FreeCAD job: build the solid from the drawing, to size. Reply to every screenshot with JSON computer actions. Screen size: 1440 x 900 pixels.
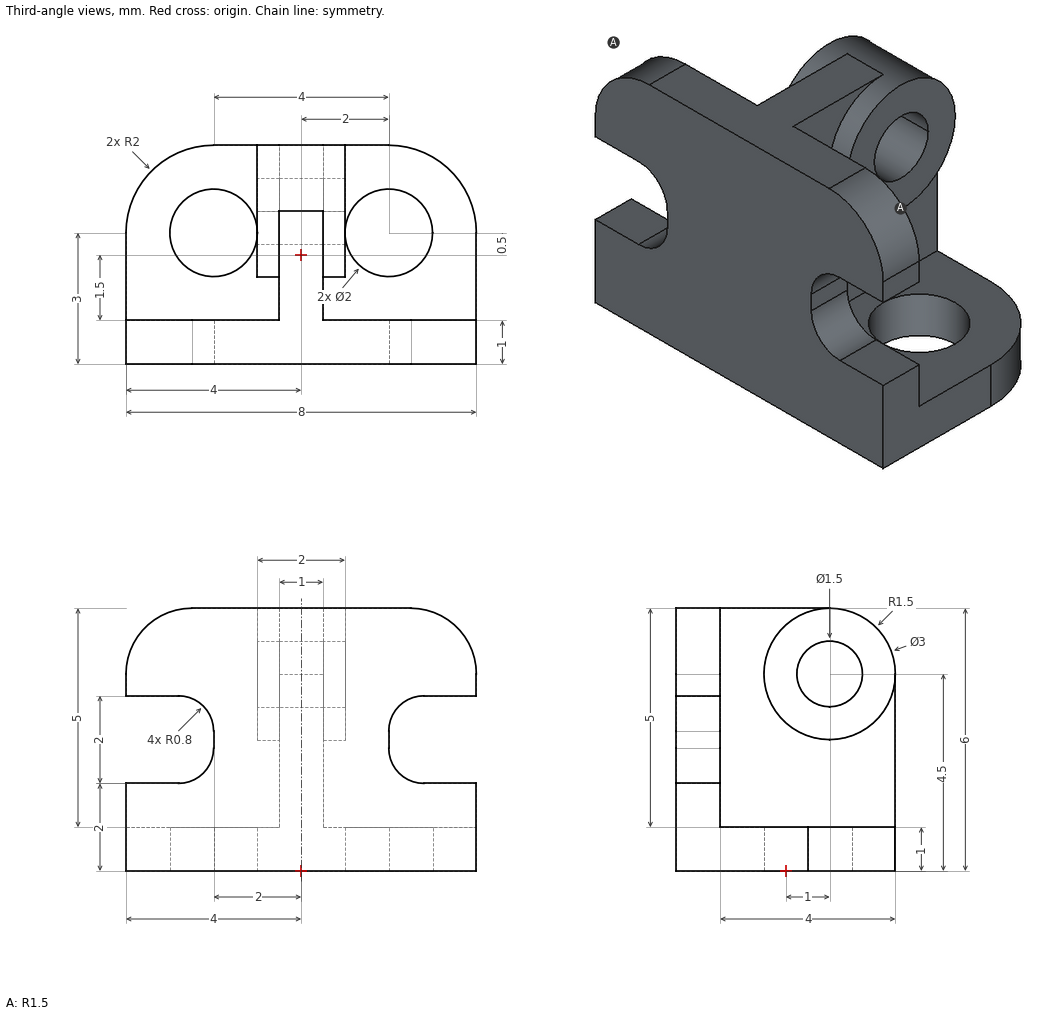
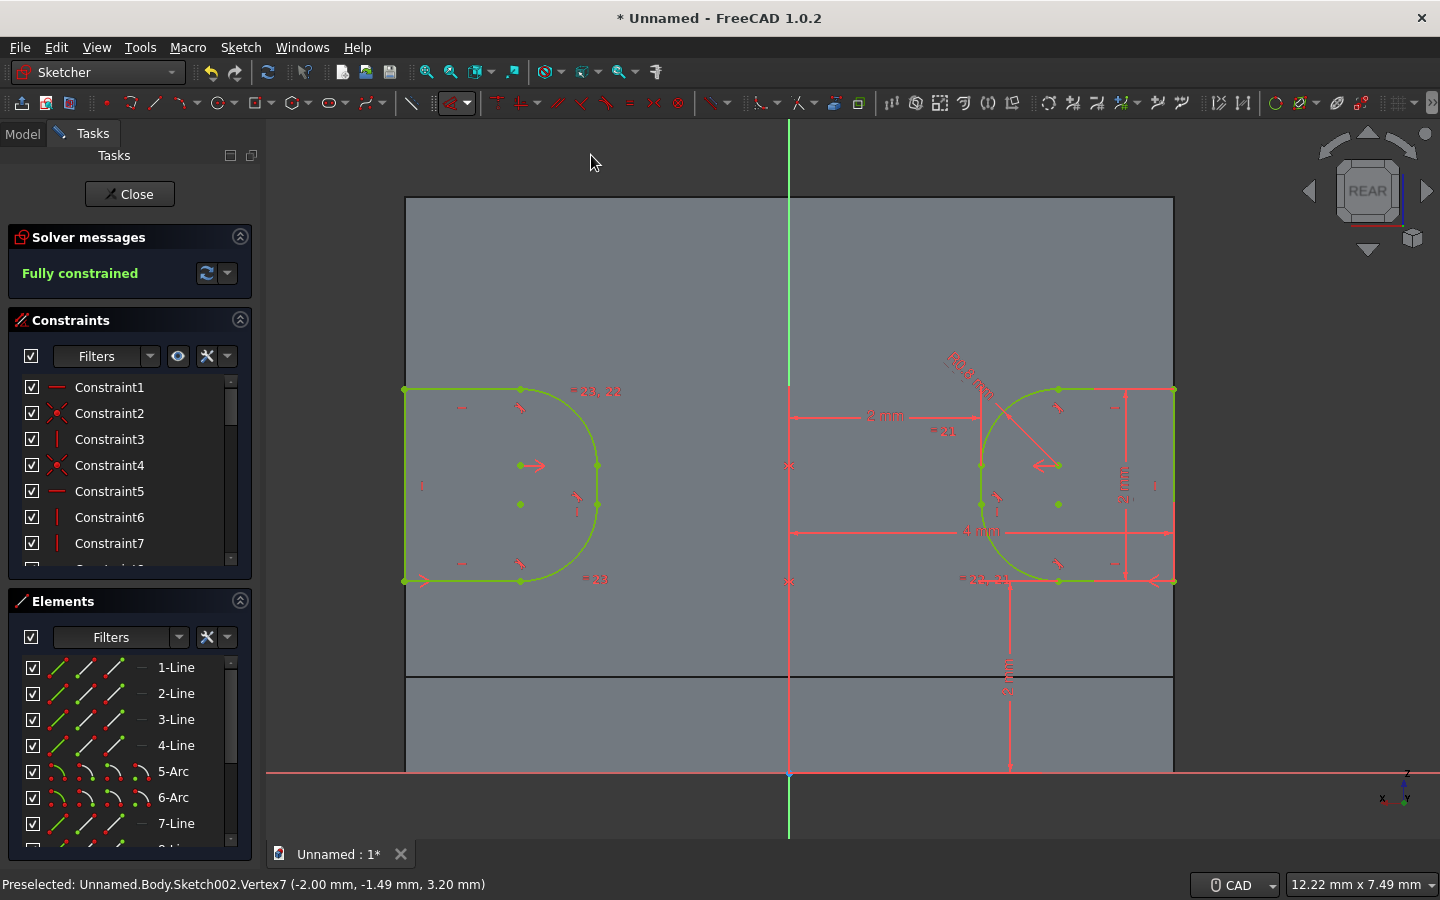
{"action": "left_click", "coordinate": [130, 194]}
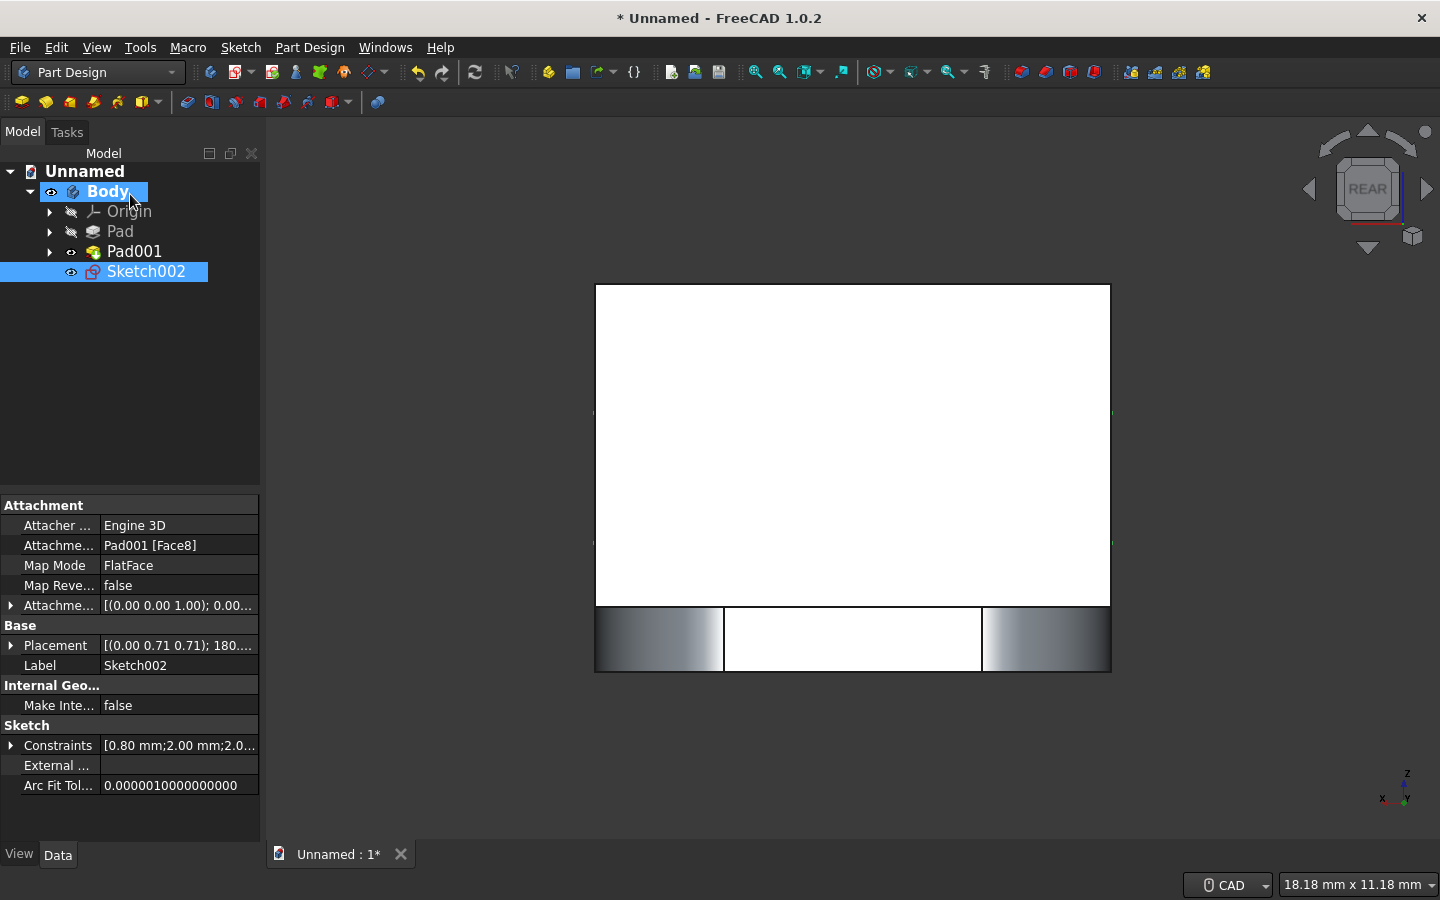
{"action": "left_click", "coordinate": [188, 102]}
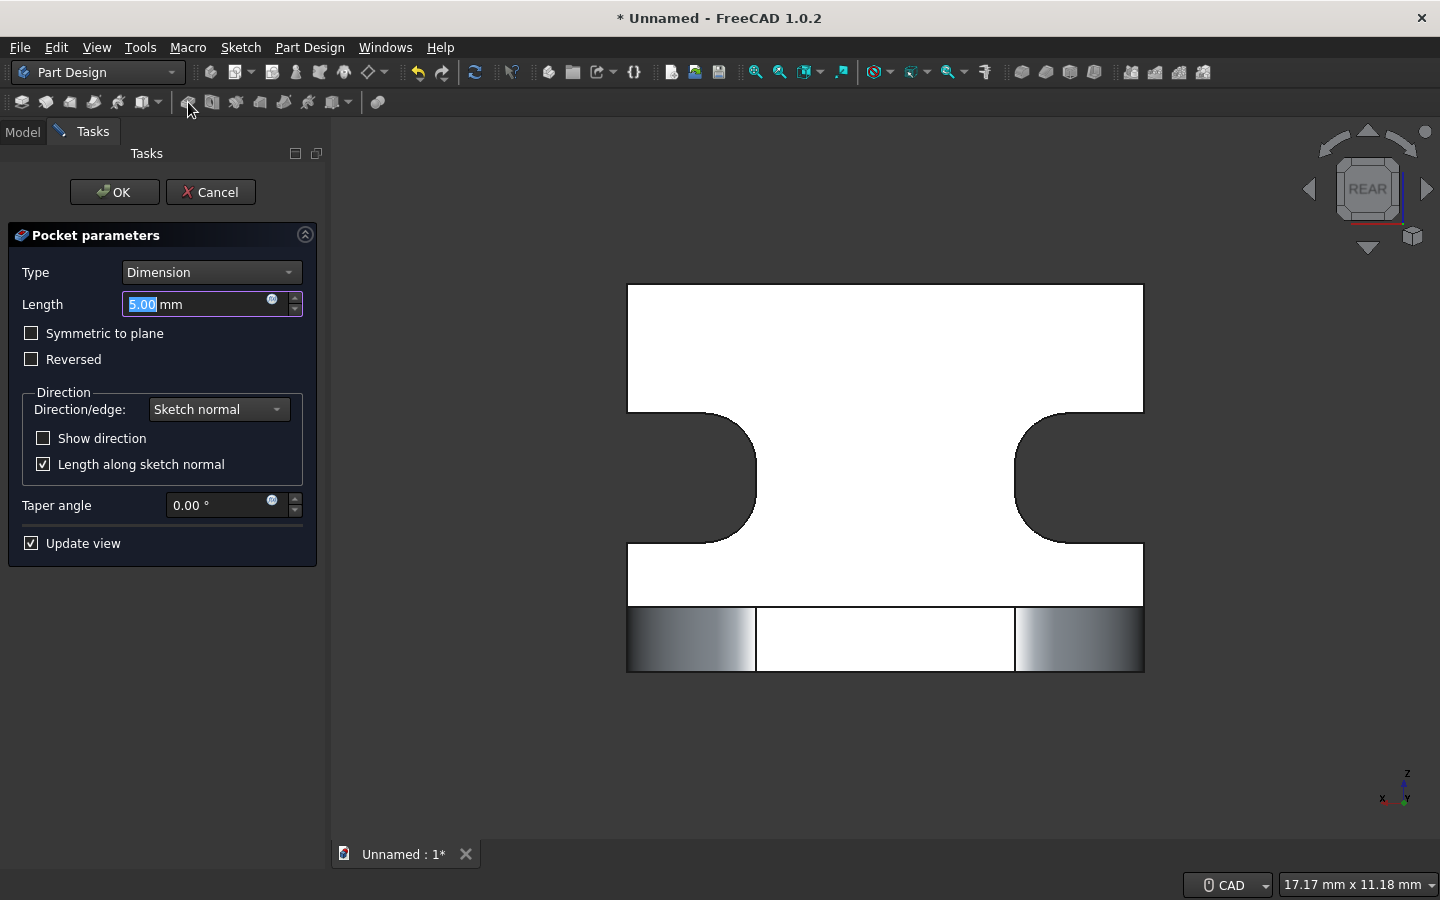
{"action": "left_click", "coordinate": [212, 272]}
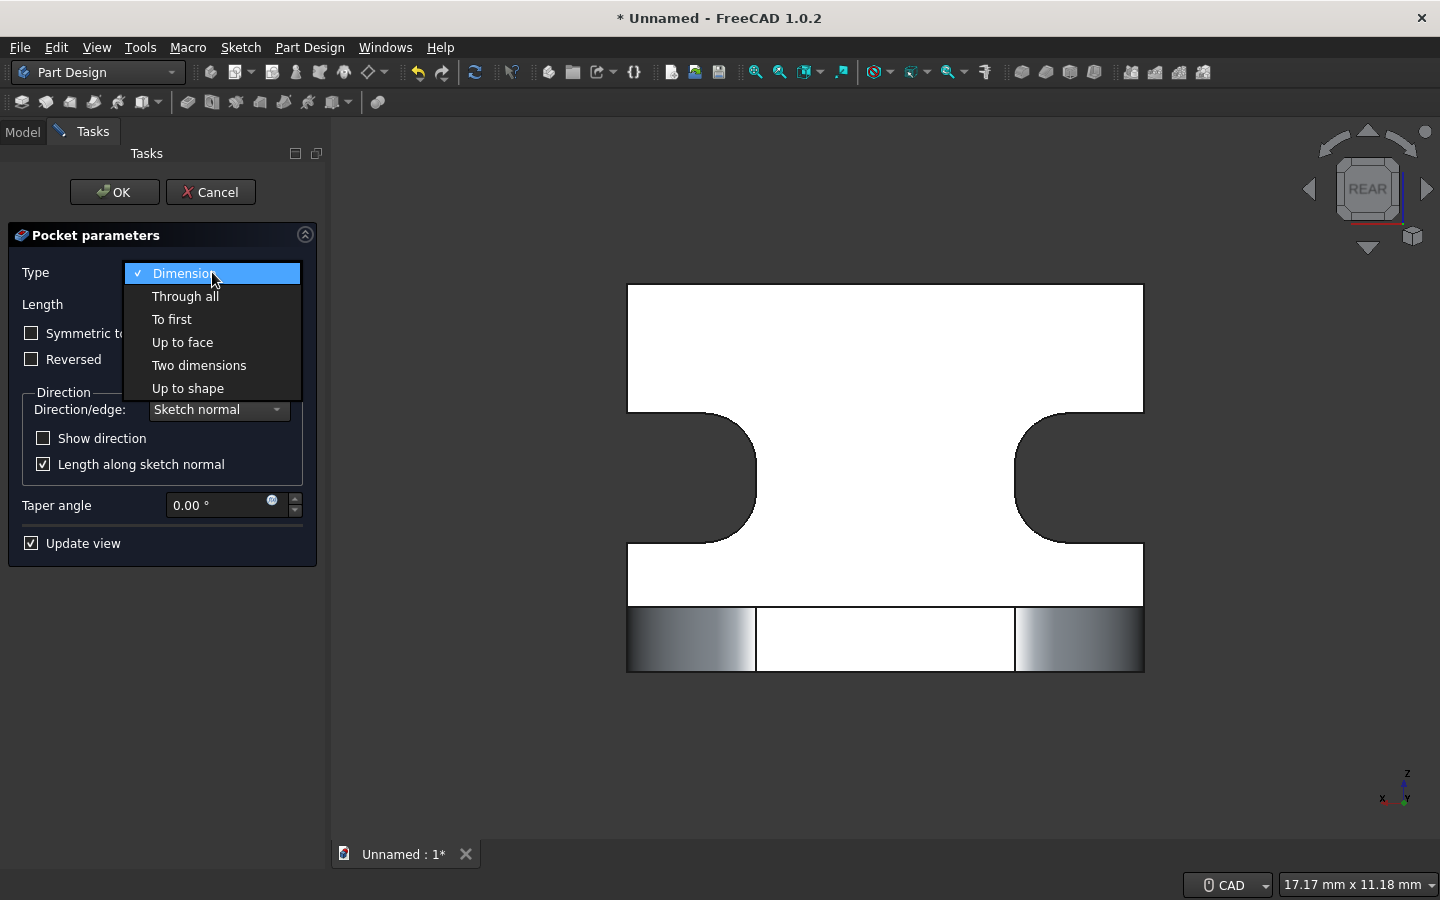
{"action": "left_click", "coordinate": [212, 296]}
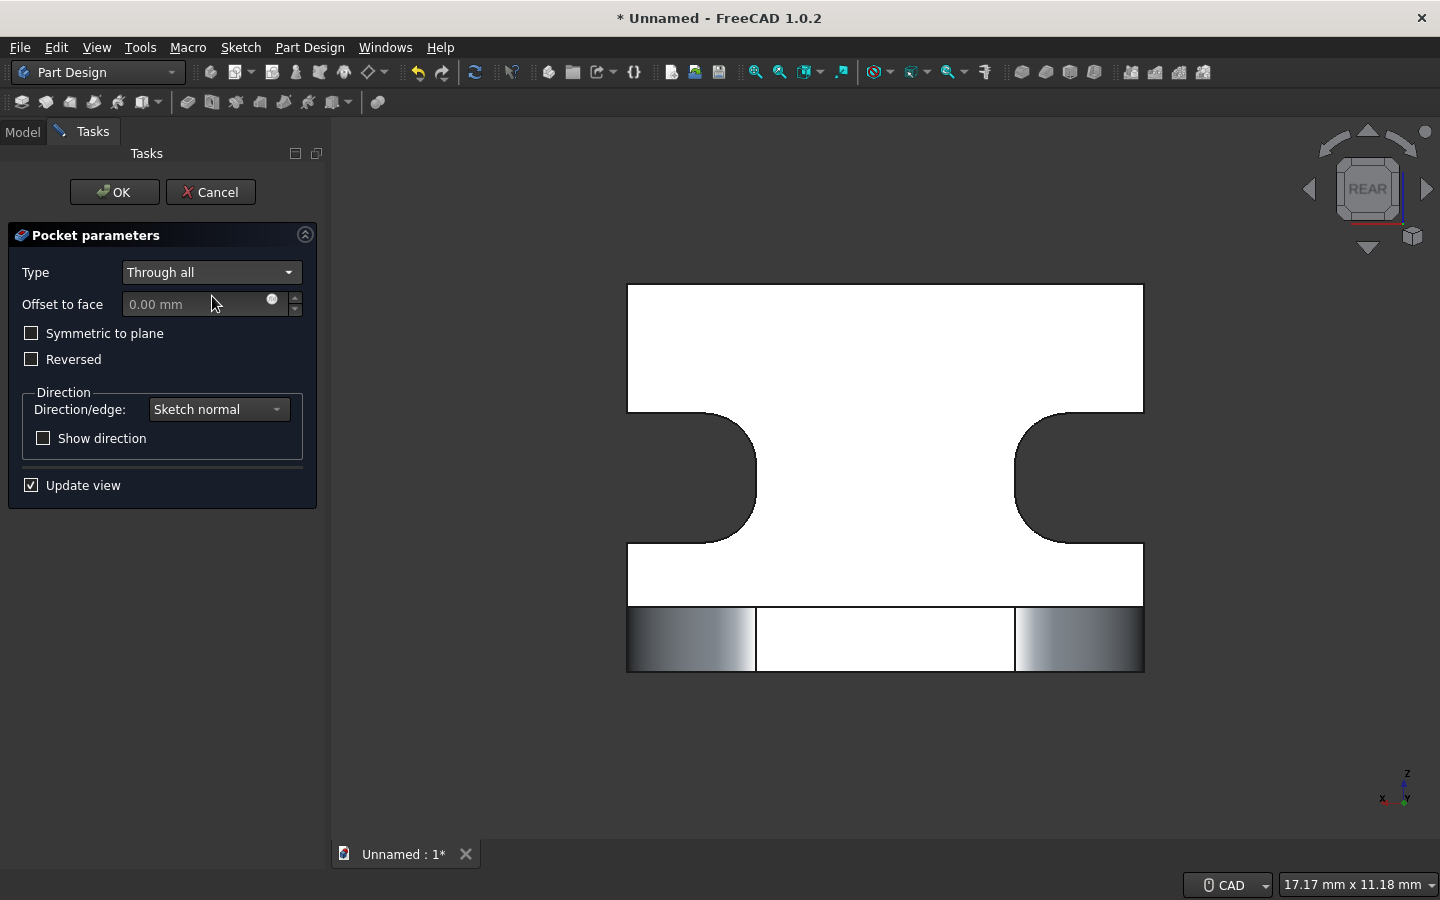
{"action": "left_click", "coordinate": [115, 192]}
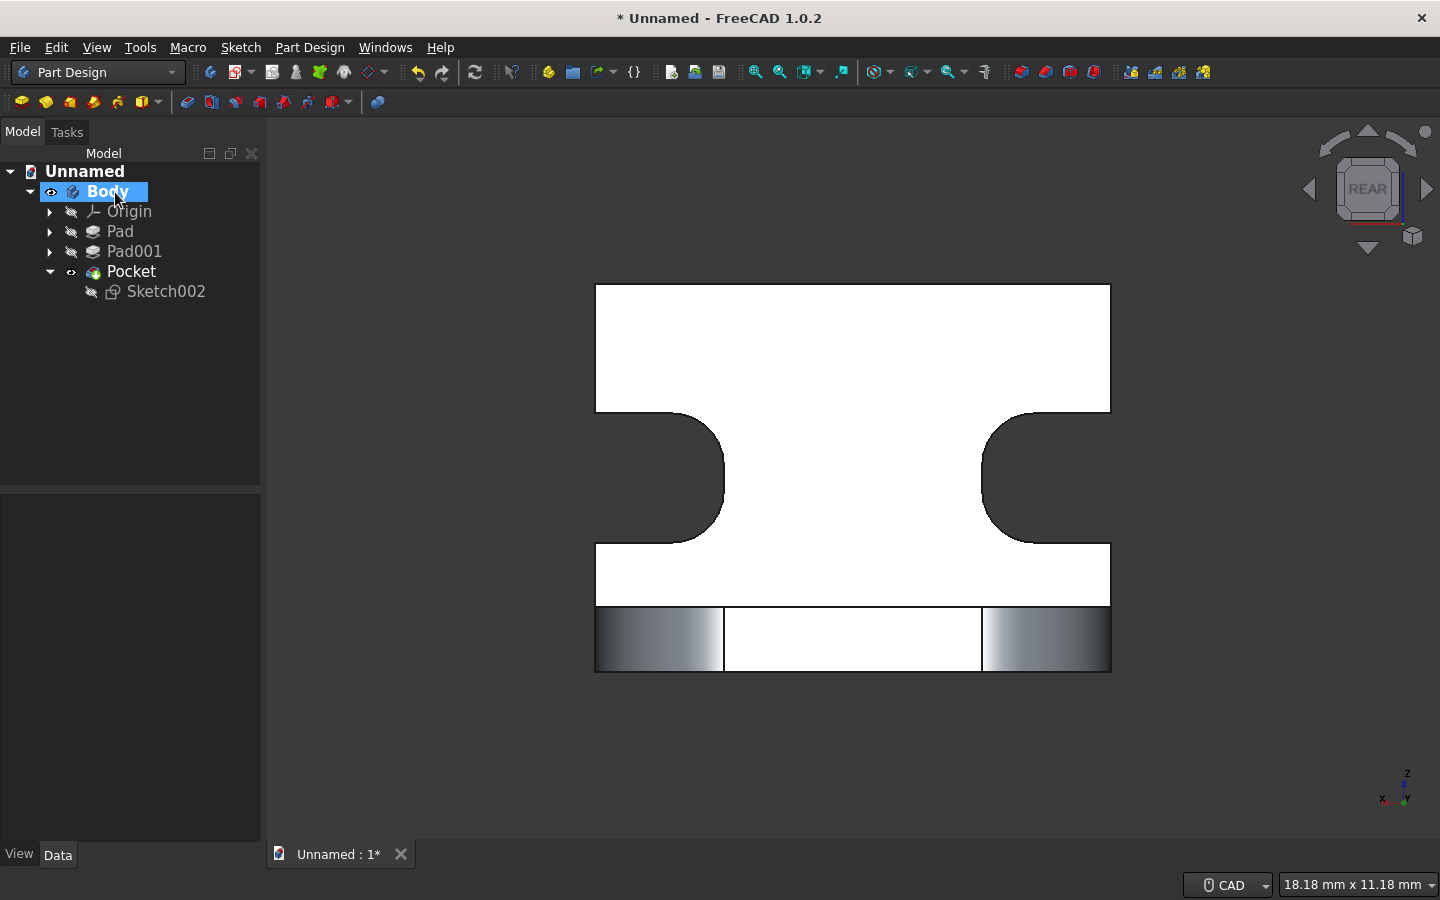
{"action": "left_click", "coordinate": [236, 72]}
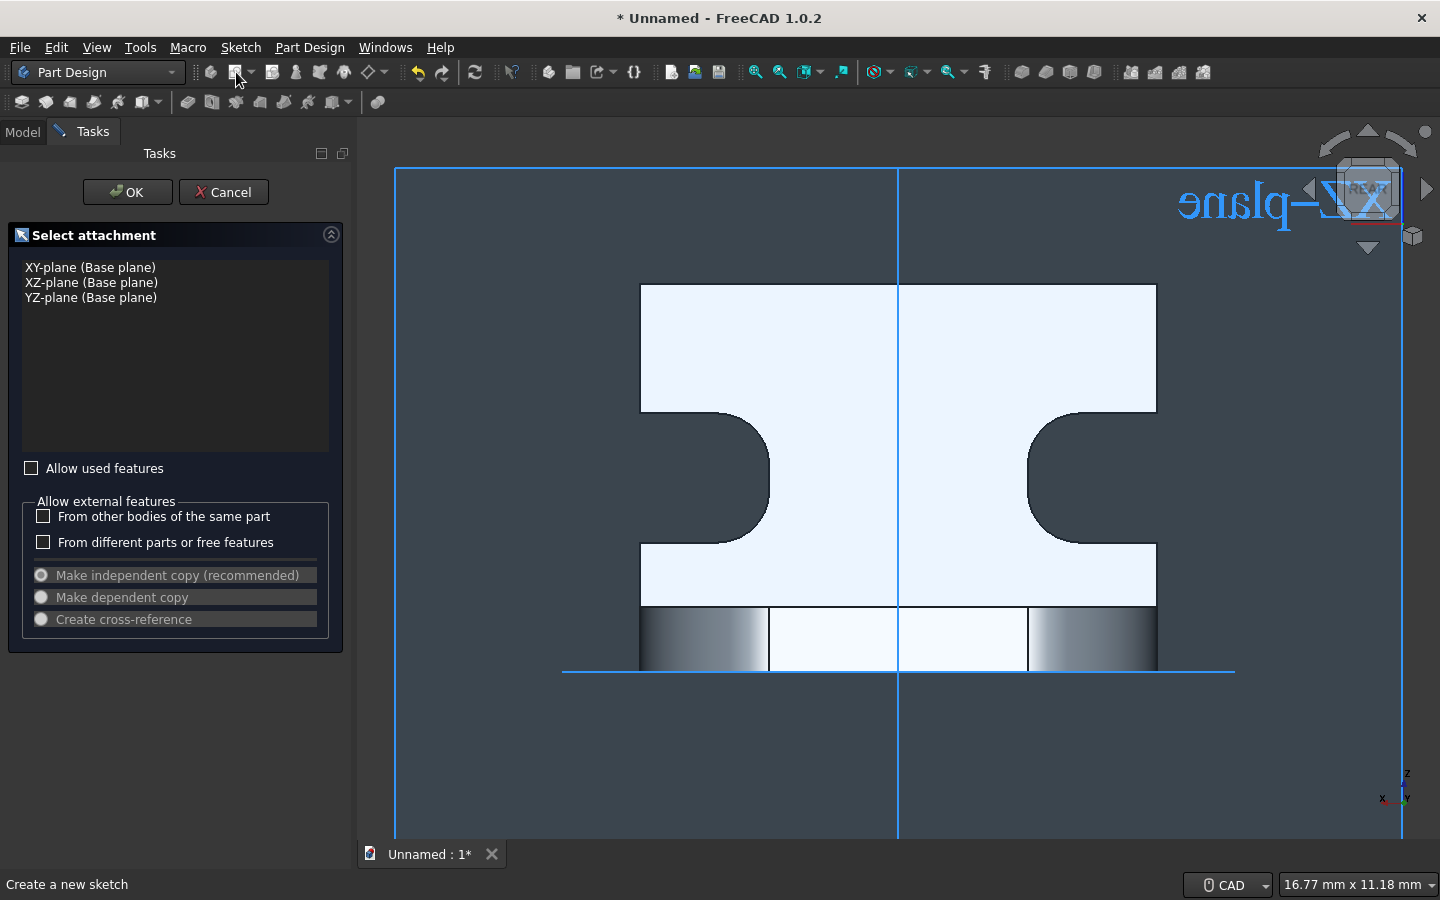
{"action": "left_click", "coordinate": [82, 298]}